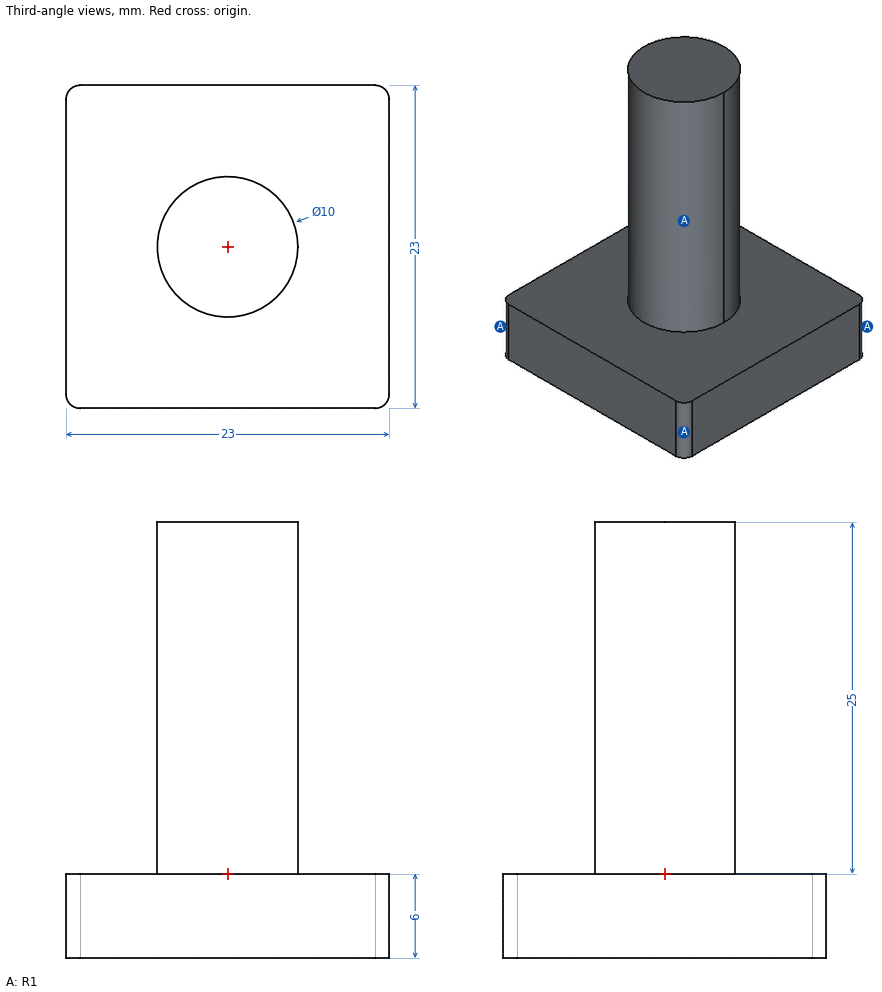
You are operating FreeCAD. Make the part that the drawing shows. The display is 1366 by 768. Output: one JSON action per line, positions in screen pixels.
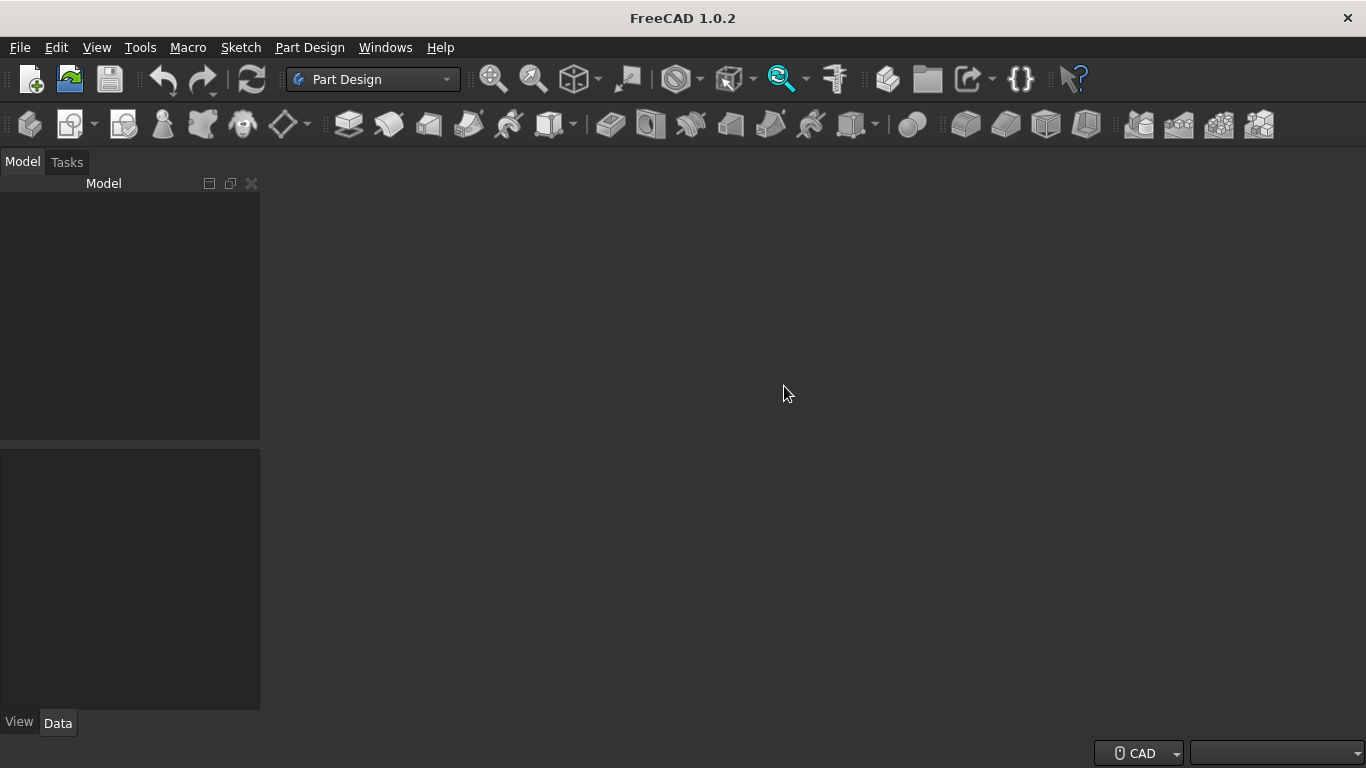
{"action": "key", "text": "ctrl+n"}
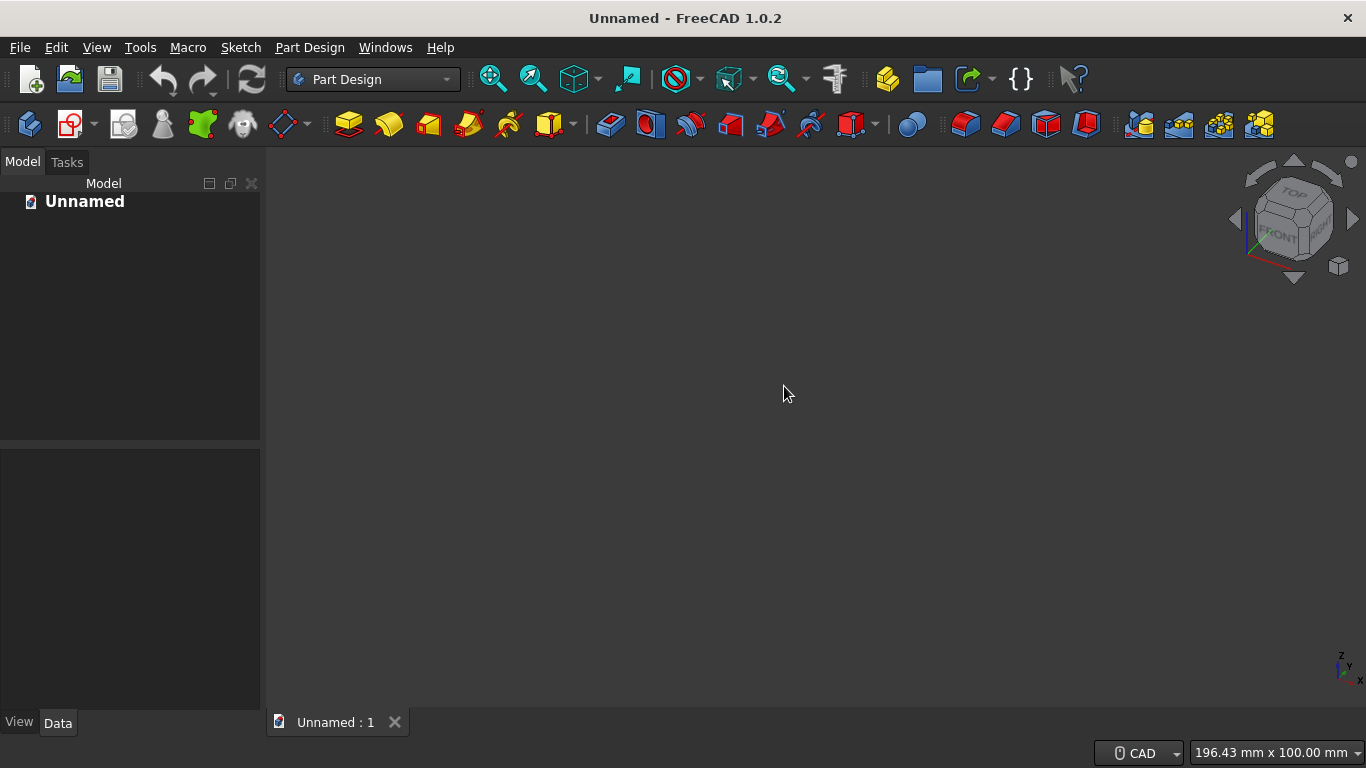
{"action": "left_click", "coordinate": [70, 124]}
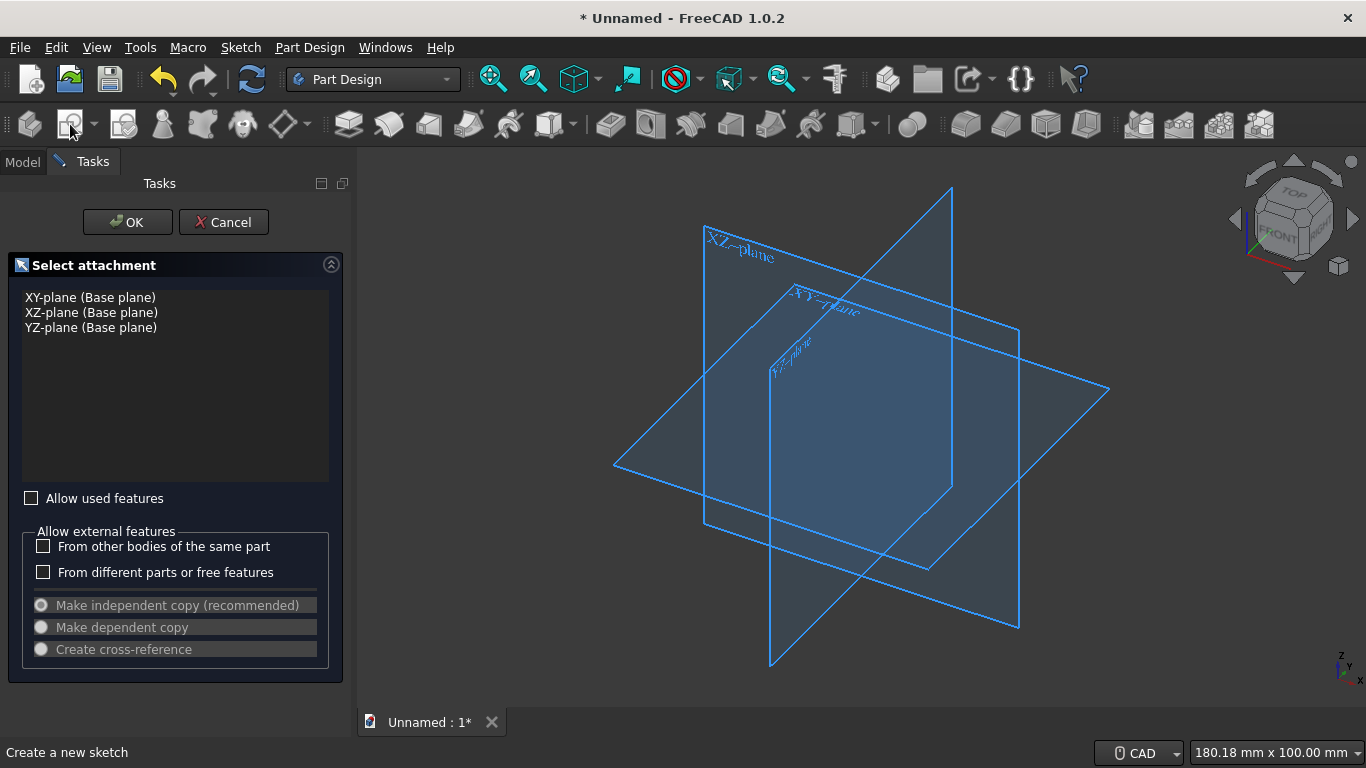
{"action": "left_click", "coordinate": [82, 298]}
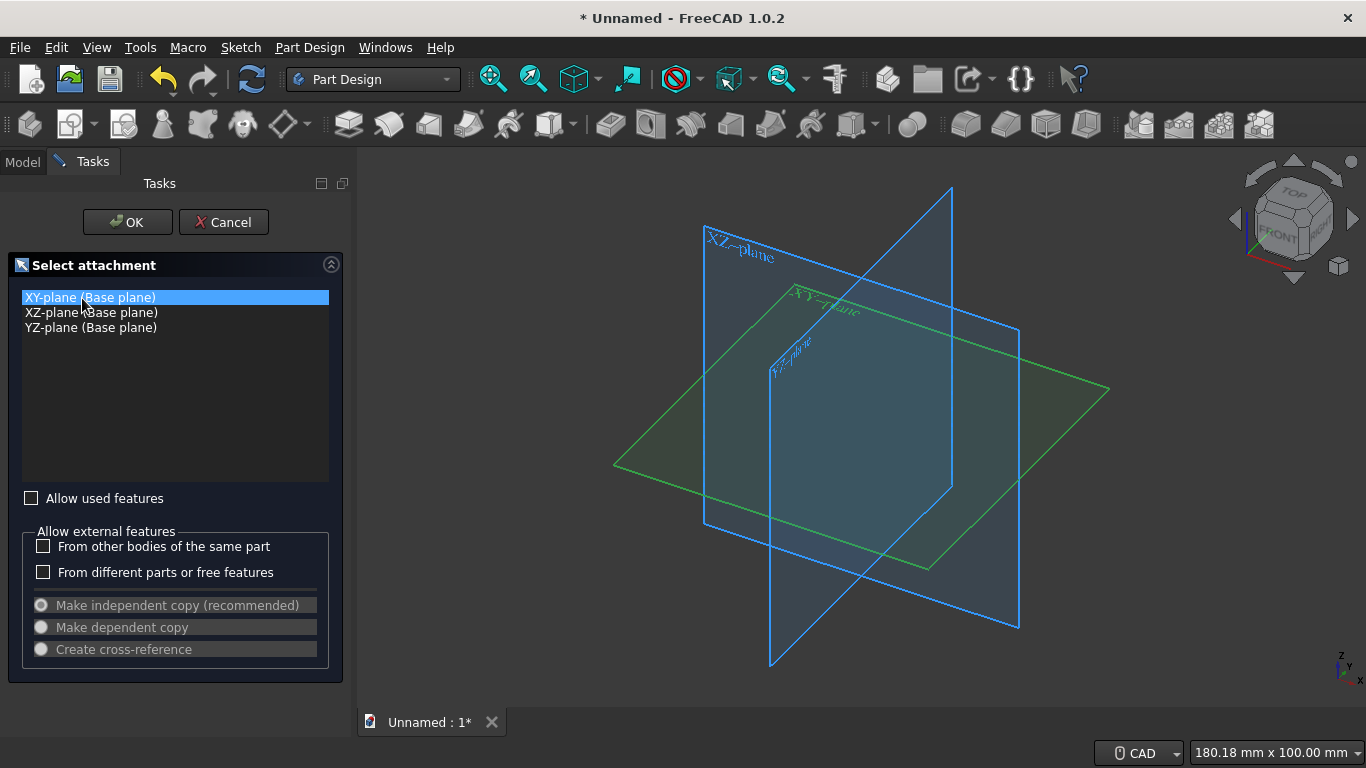
{"action": "left_click", "coordinate": [128, 222]}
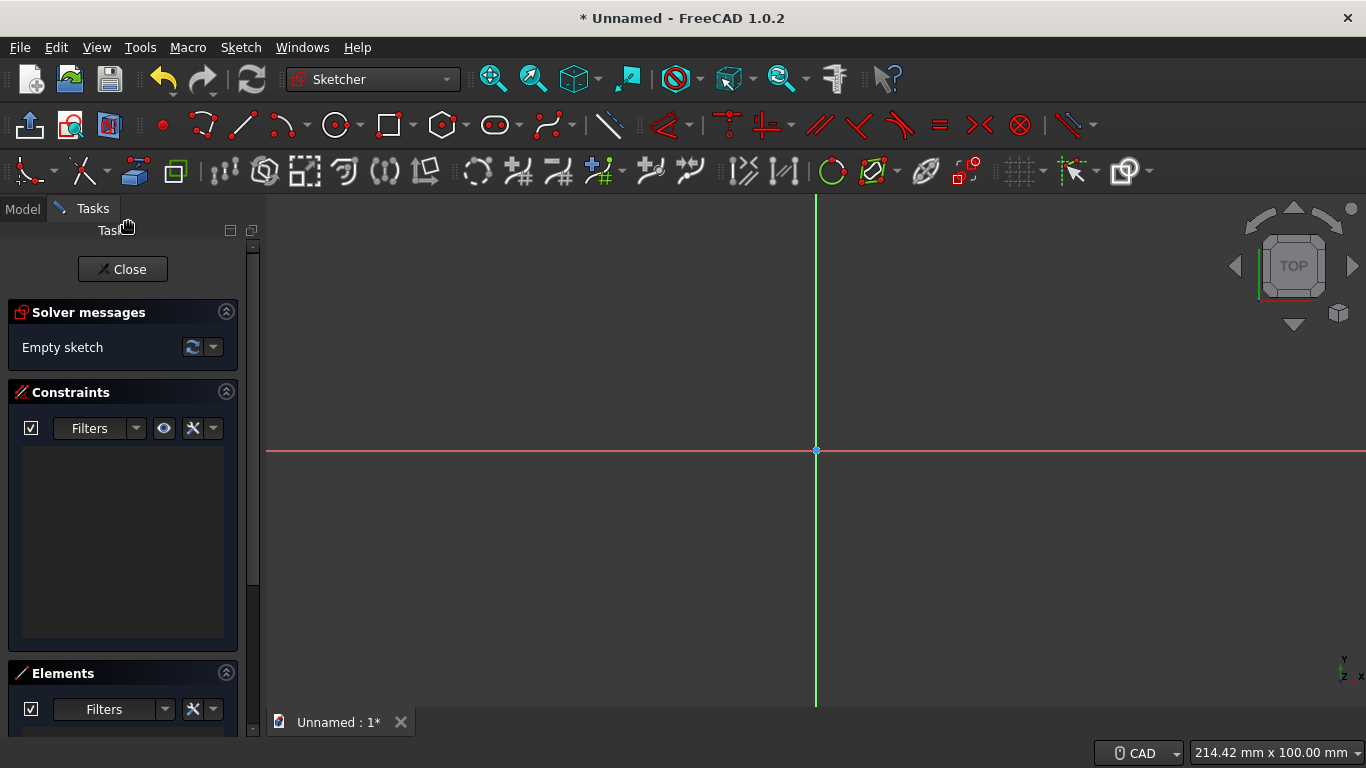
{"action": "scroll", "coordinate": [830, 451], "scroll_direction": "up", "scroll_amount": 9}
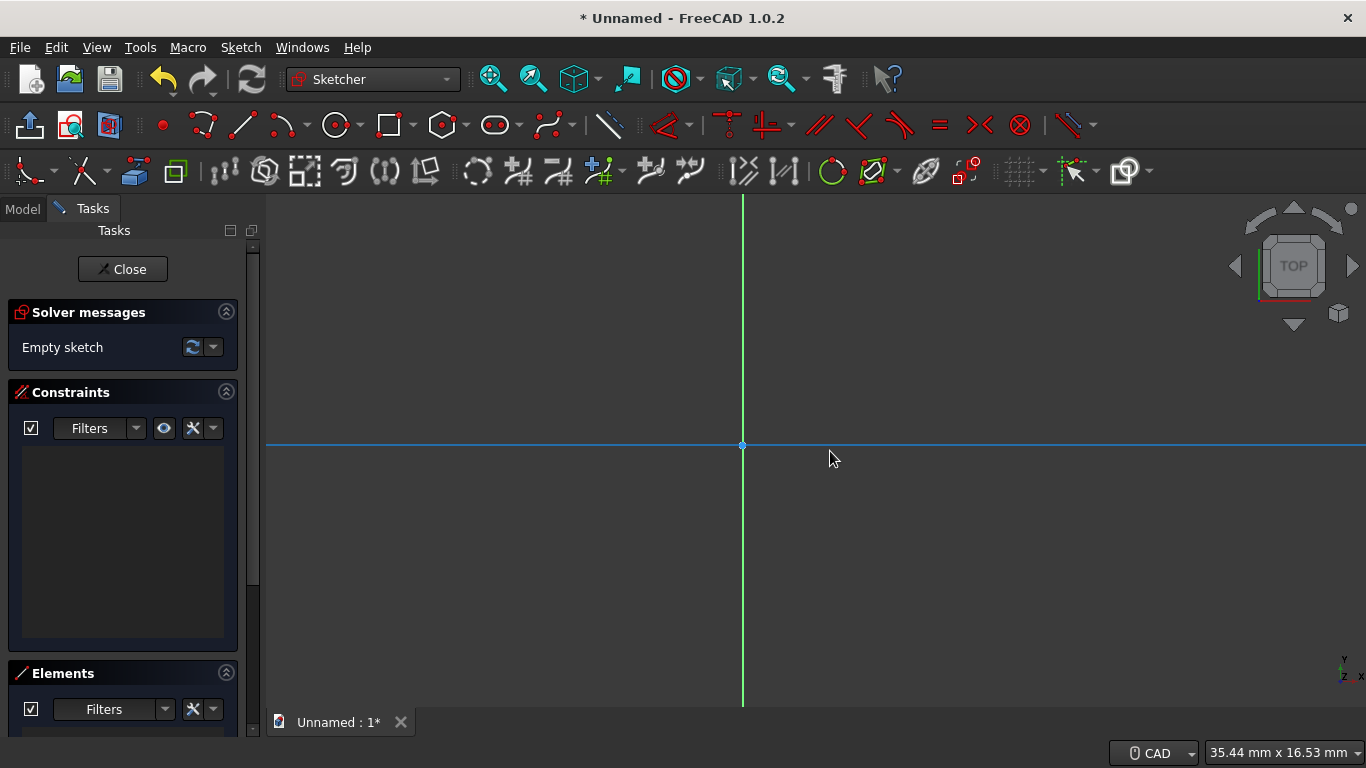
{"action": "left_click", "coordinate": [336, 126]}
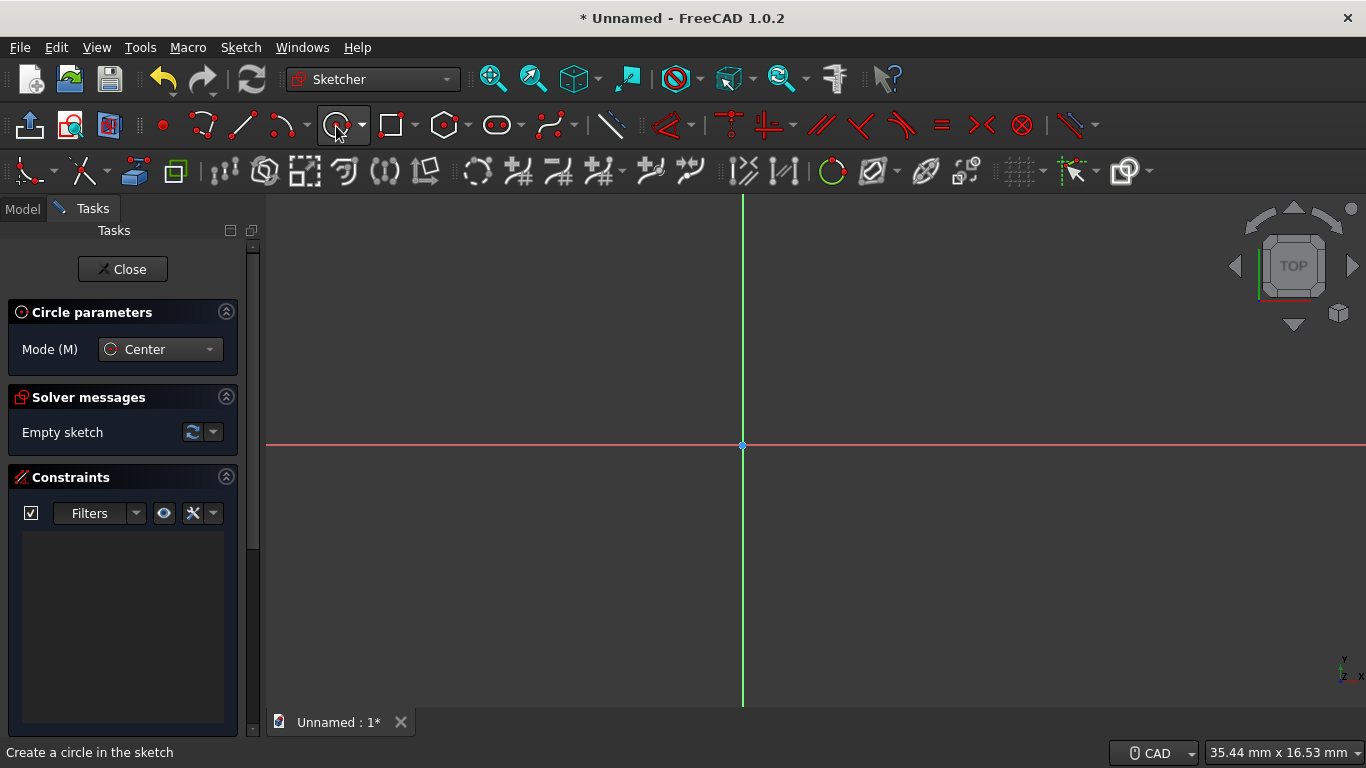
{"action": "left_click", "coordinate": [743, 445]}
{"action": "mouse_move", "coordinate": [852, 336]}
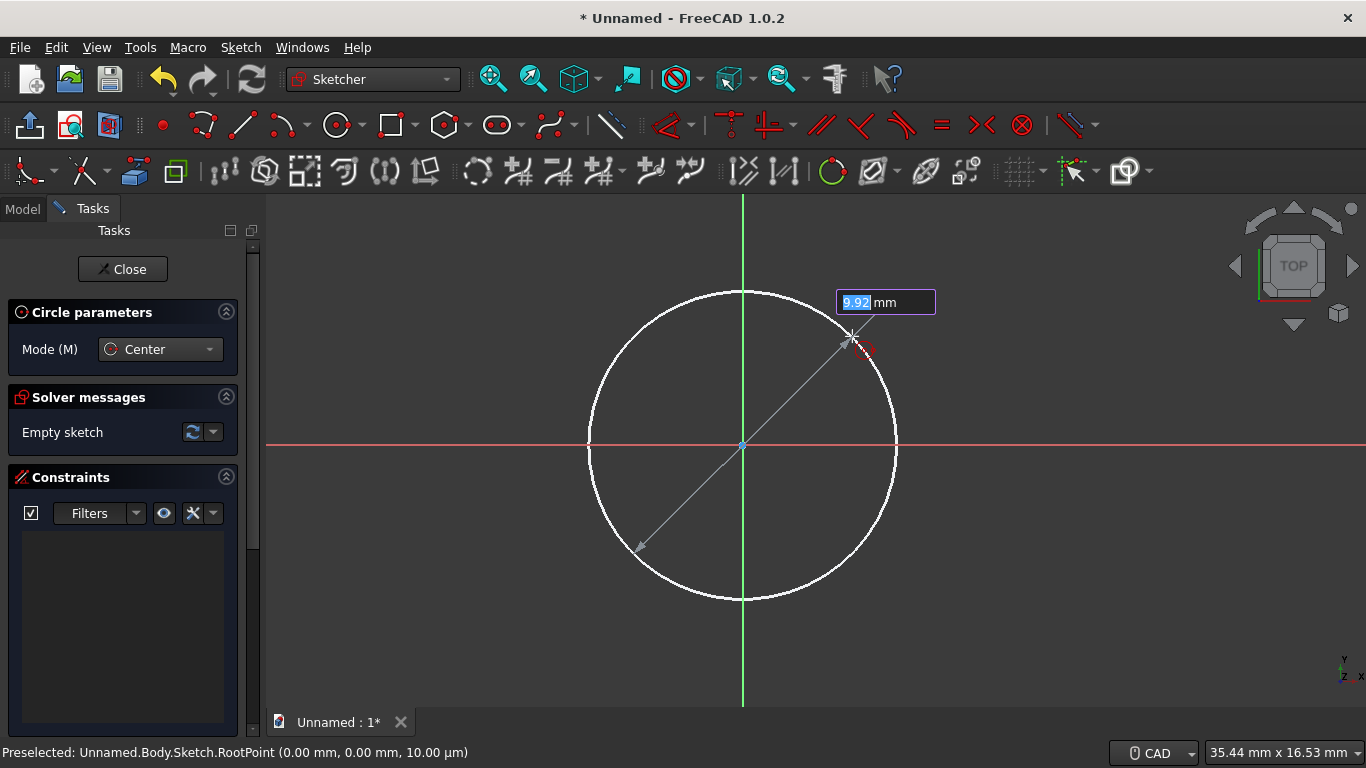
{"action": "type", "text": "10"}
{"action": "key", "text": "Return"}
{"action": "key", "text": "Escape"}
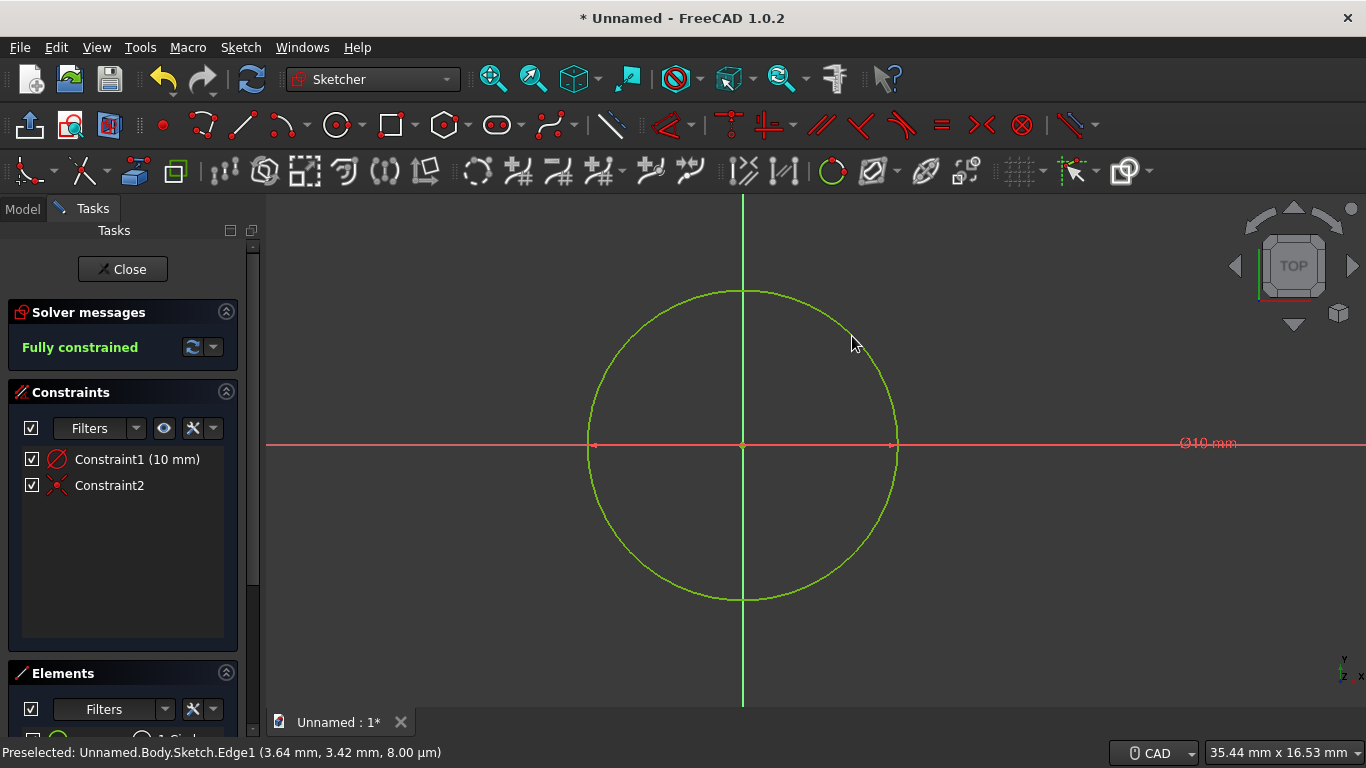
{"action": "left_click", "coordinate": [123, 269]}